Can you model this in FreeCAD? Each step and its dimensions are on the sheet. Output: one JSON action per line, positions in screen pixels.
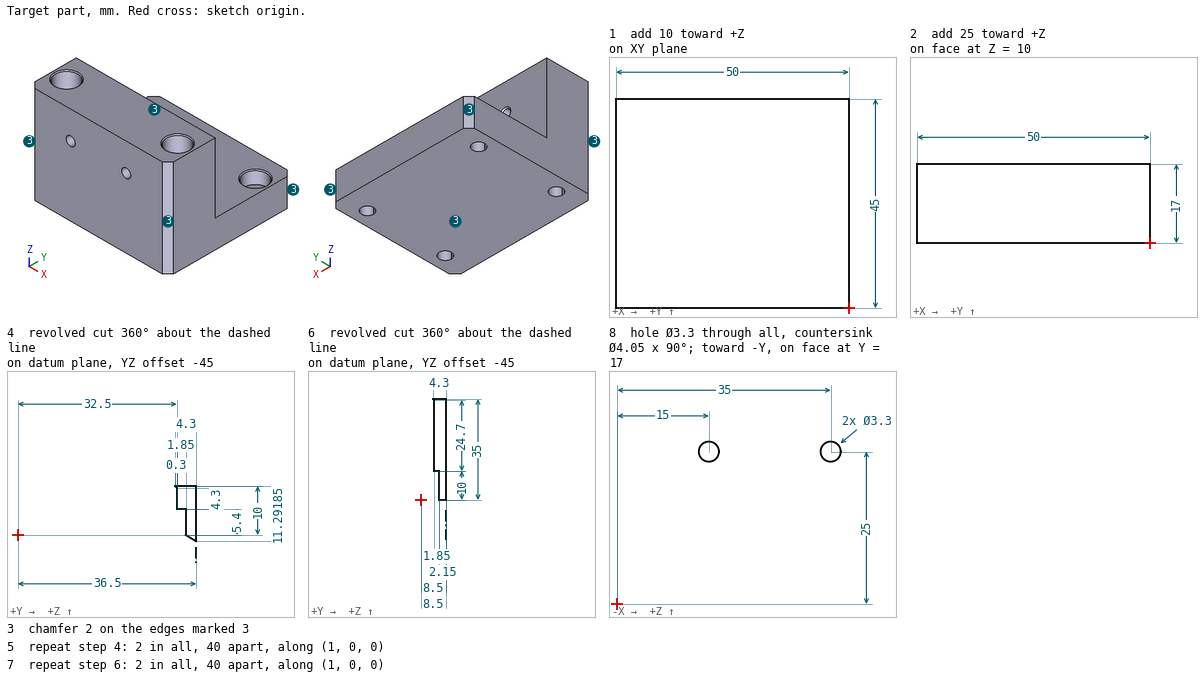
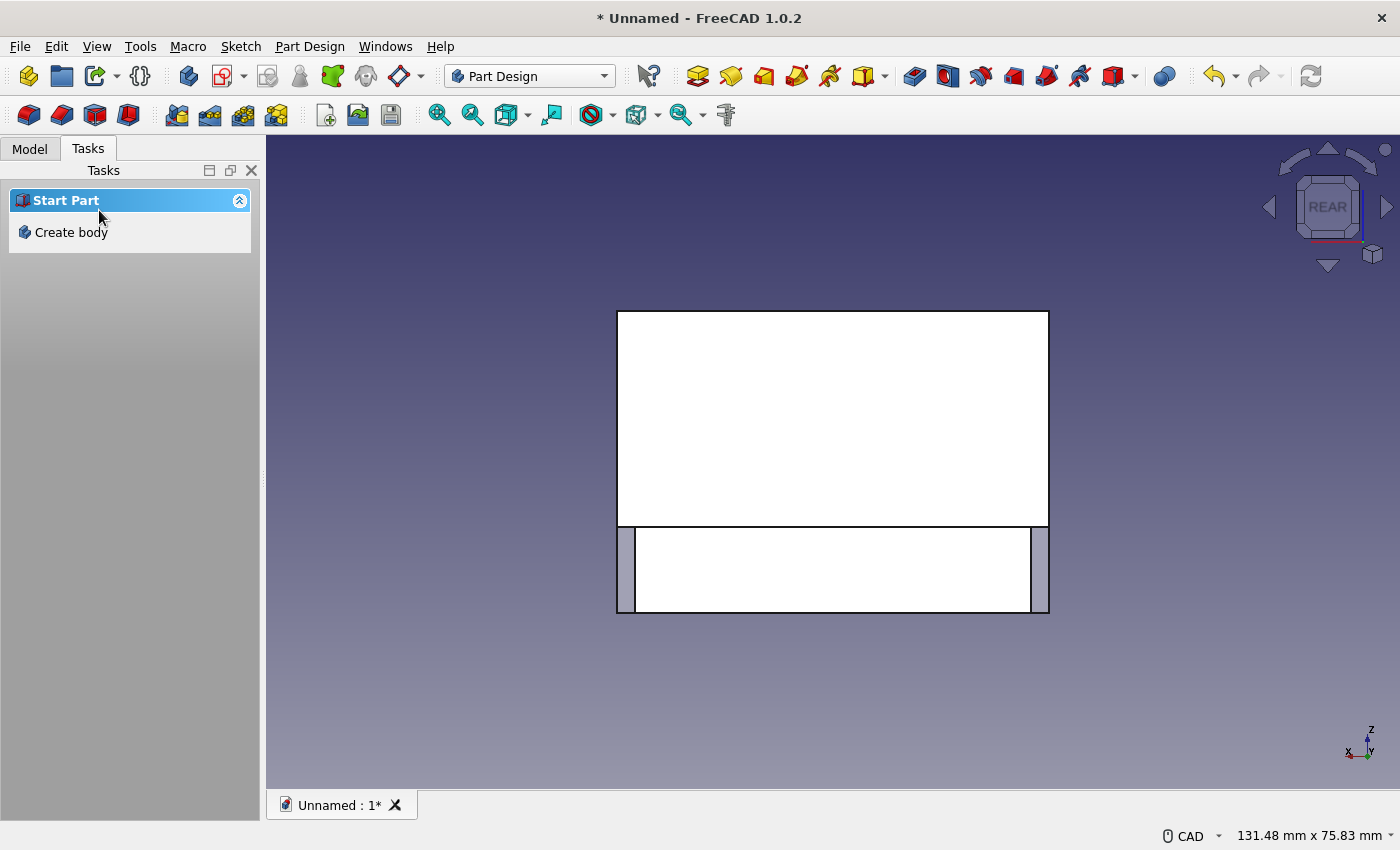
{"action": "left_click", "coordinate": [30, 148]}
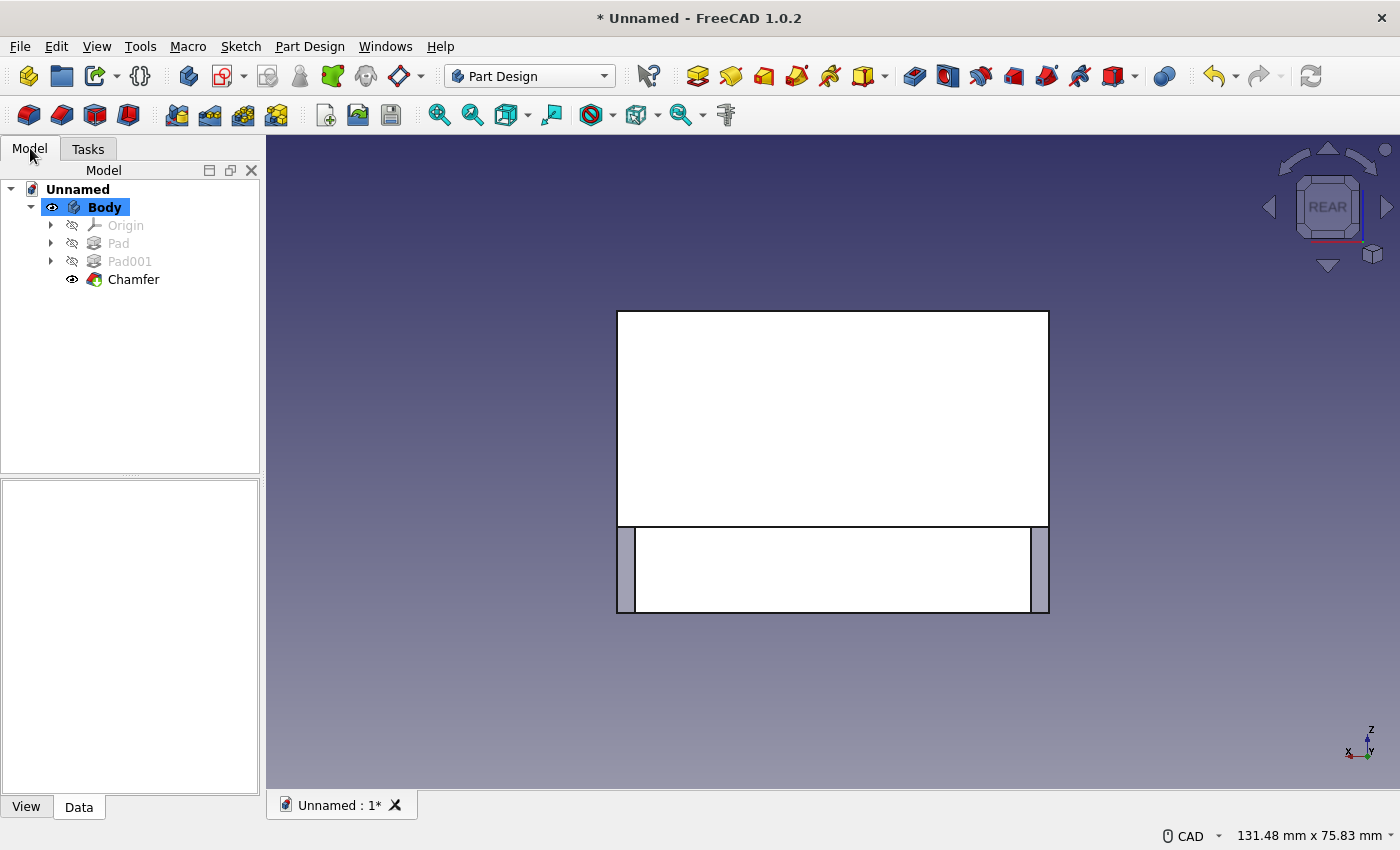
{"action": "left_click", "coordinate": [51, 225]}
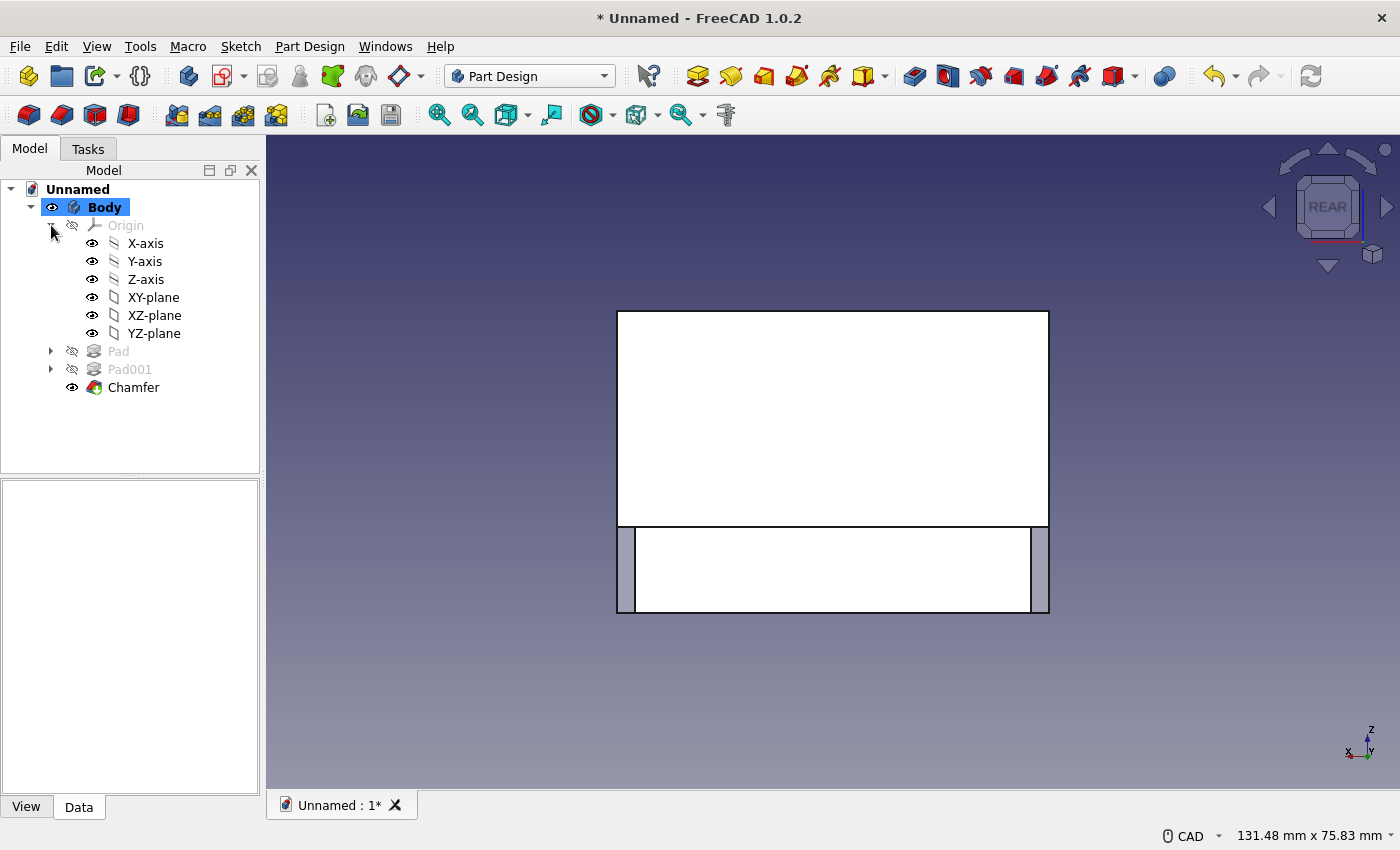
{"action": "left_click", "coordinate": [137, 333]}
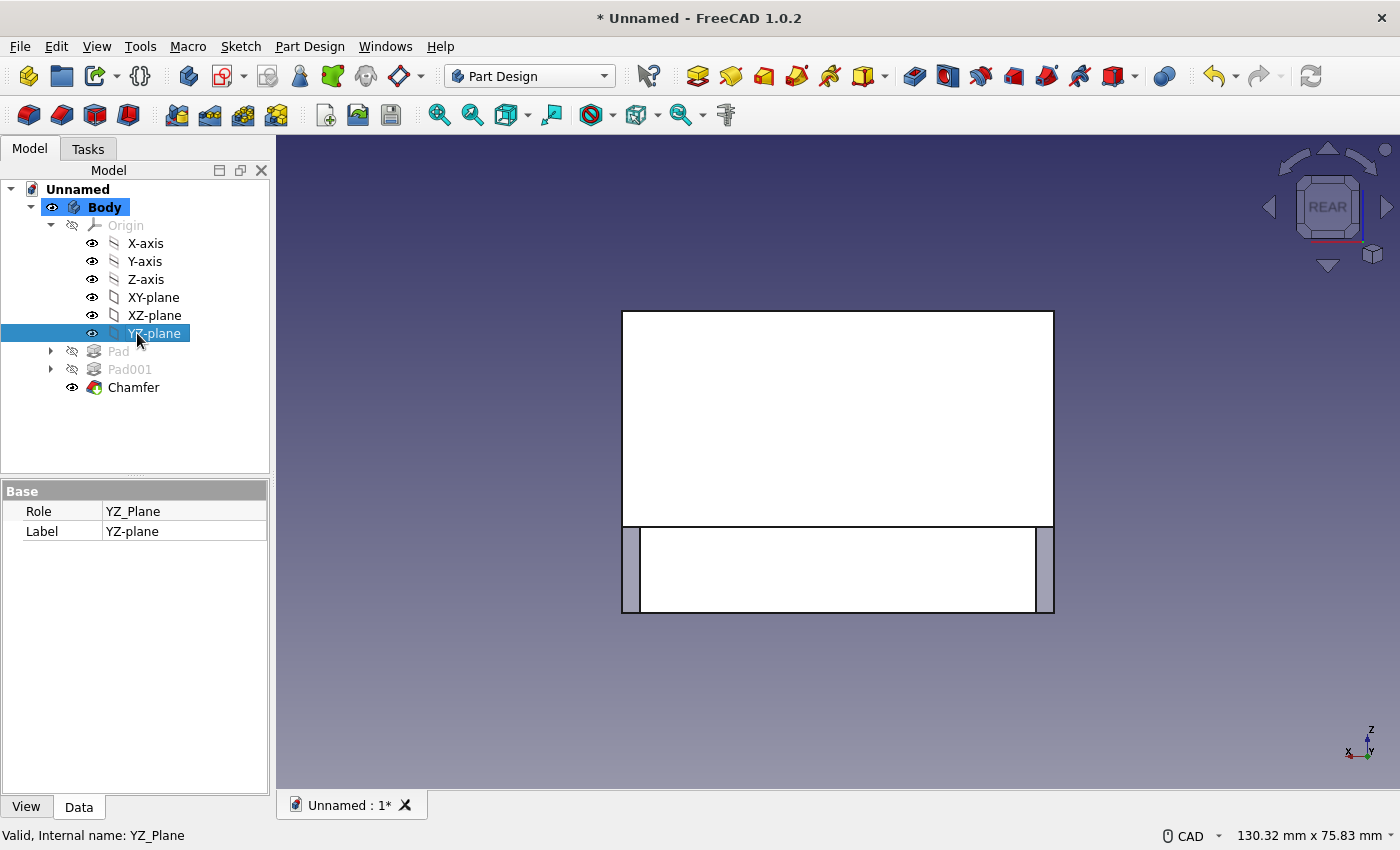
{"action": "left_click", "coordinate": [398, 76]}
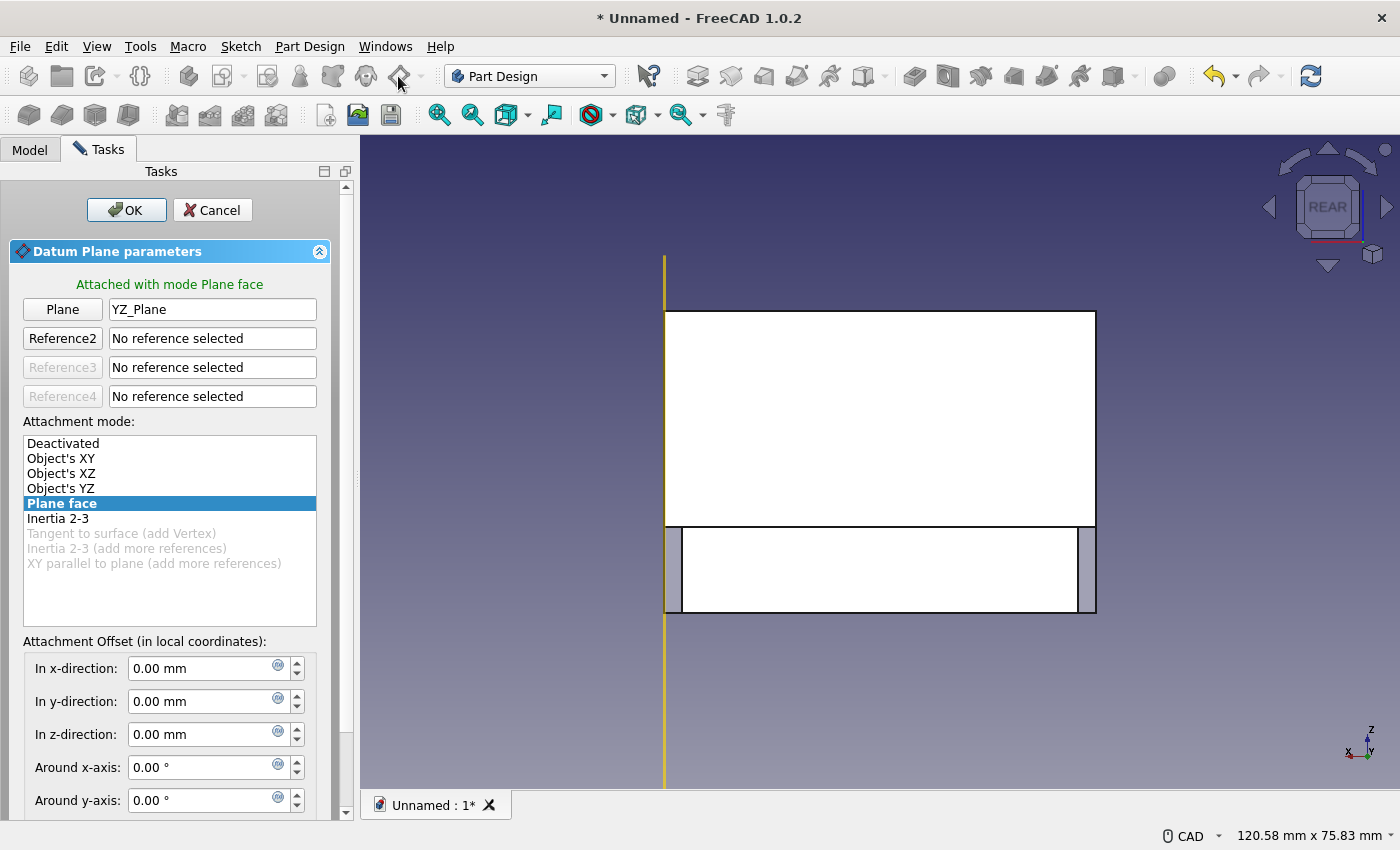
{"action": "triple_click", "coordinate": [210, 734]}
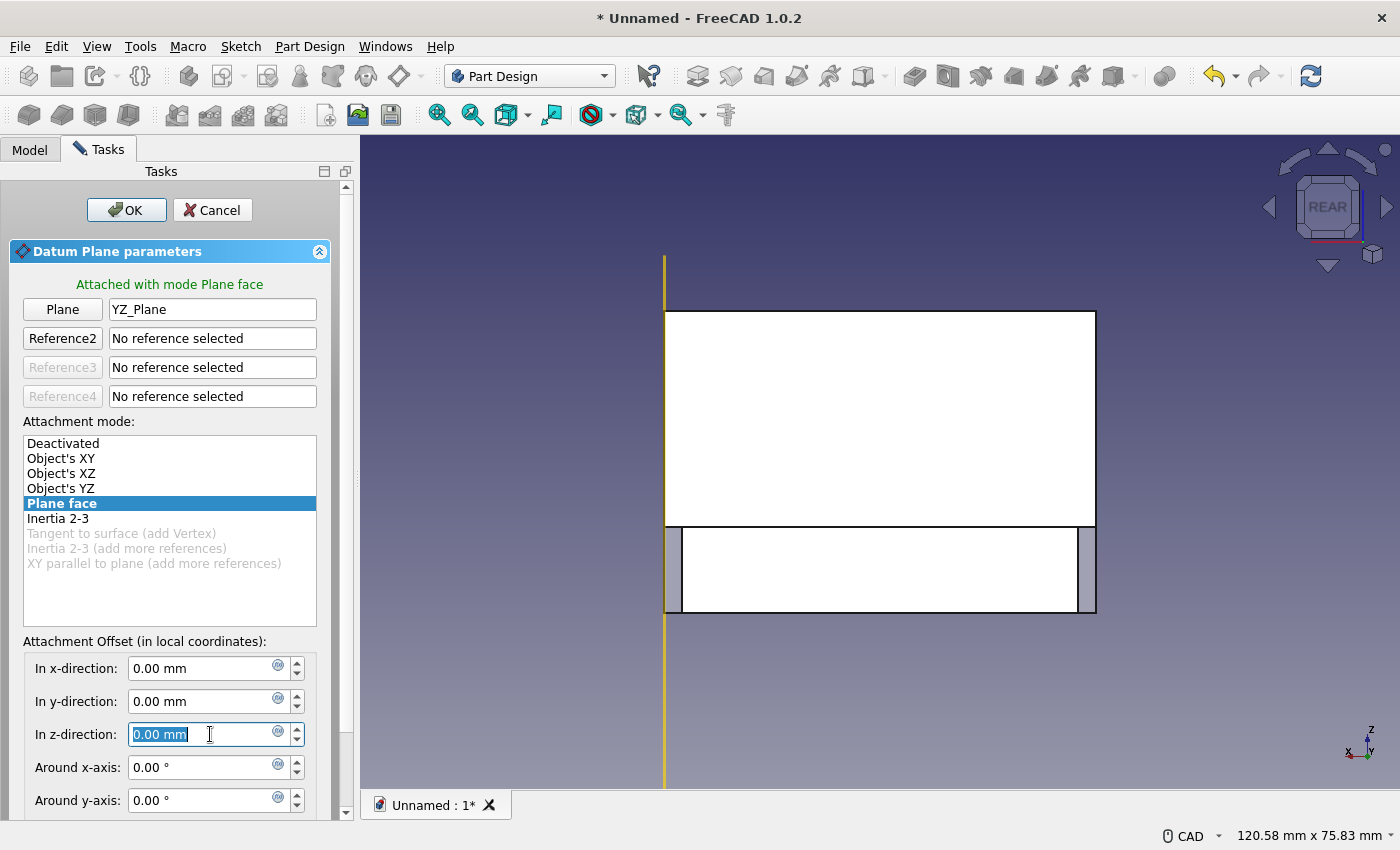
{"action": "type", "text": "-45"}
{"action": "key", "text": "Tab"}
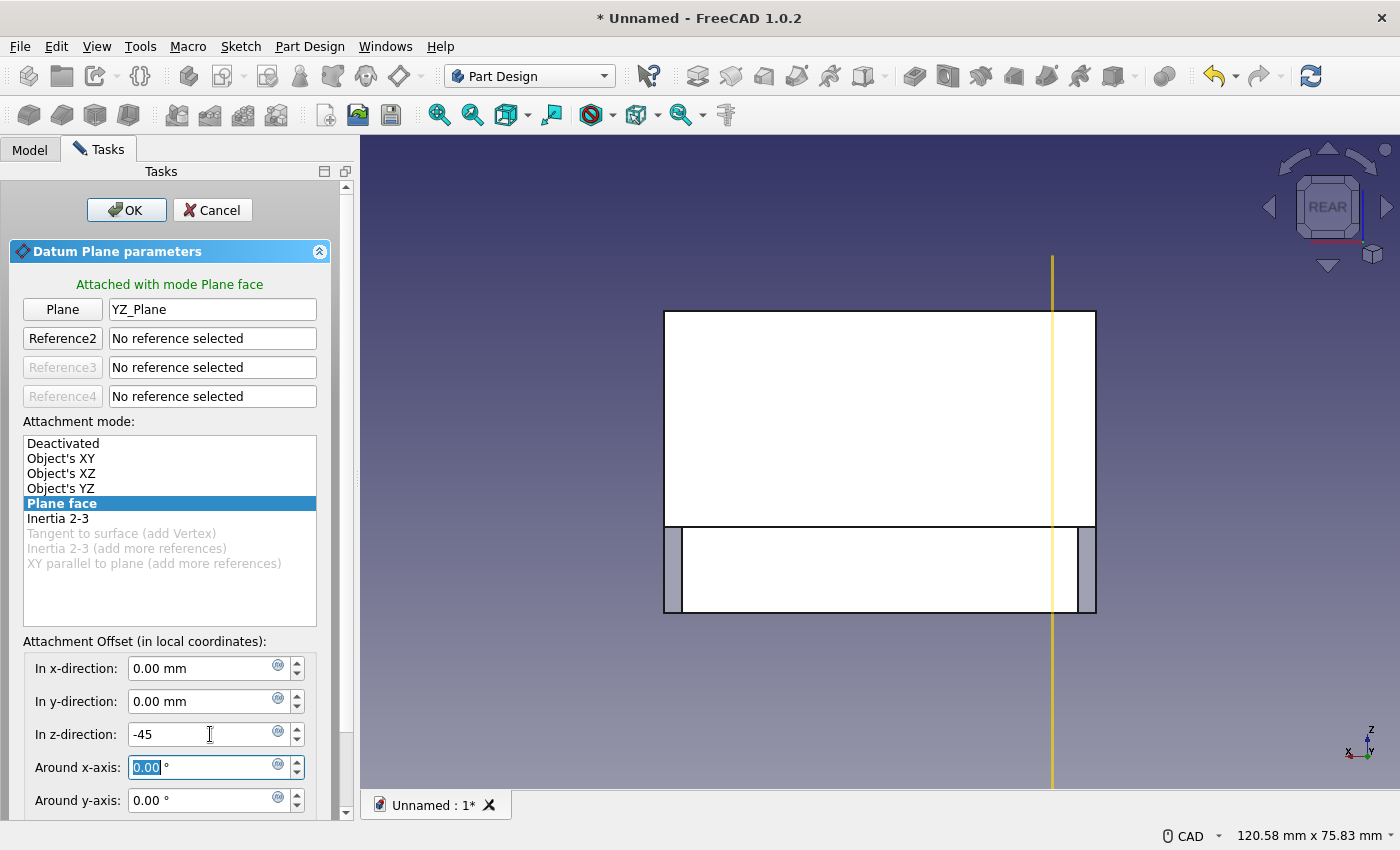
{"action": "left_click", "coordinate": [127, 210]}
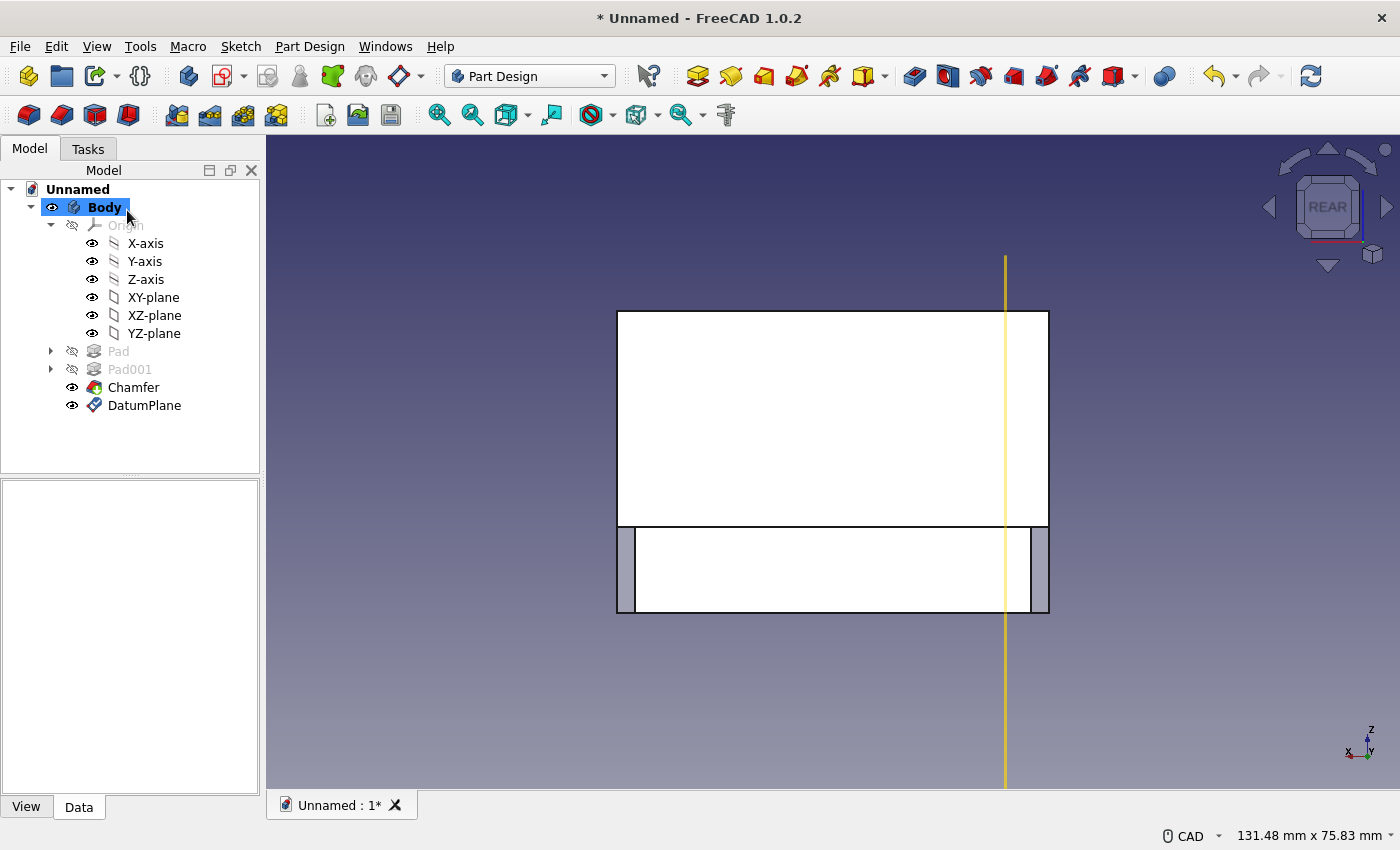
{"action": "left_click", "coordinate": [117, 405]}